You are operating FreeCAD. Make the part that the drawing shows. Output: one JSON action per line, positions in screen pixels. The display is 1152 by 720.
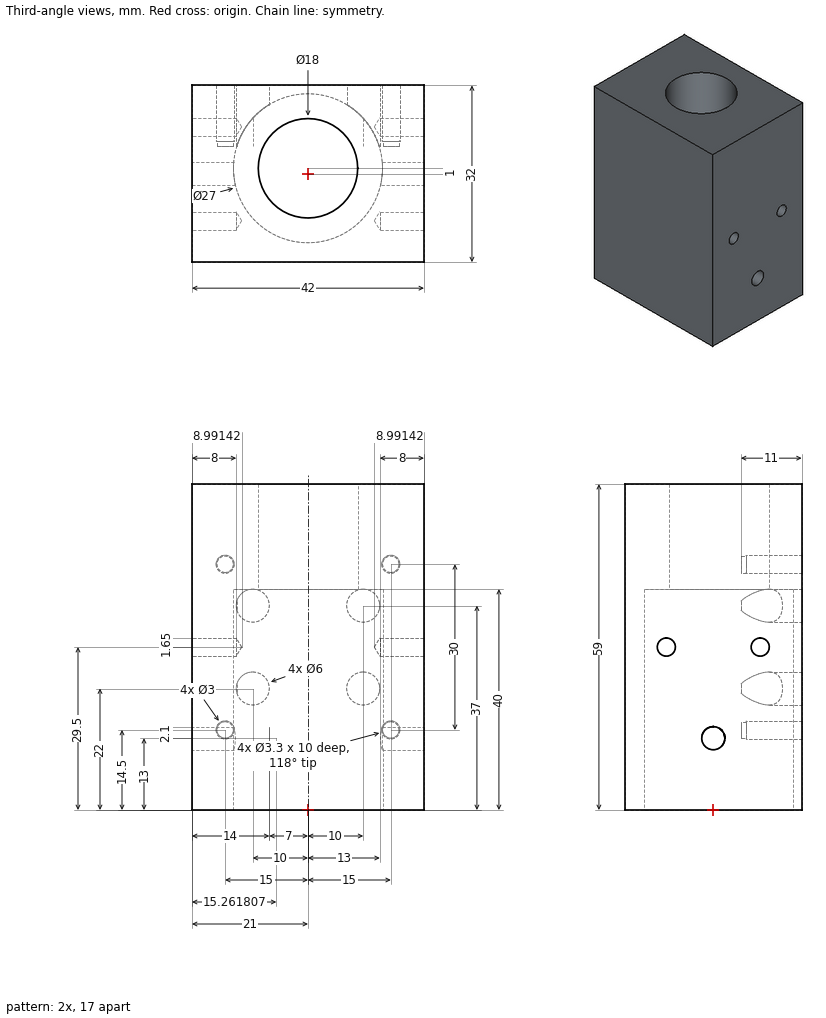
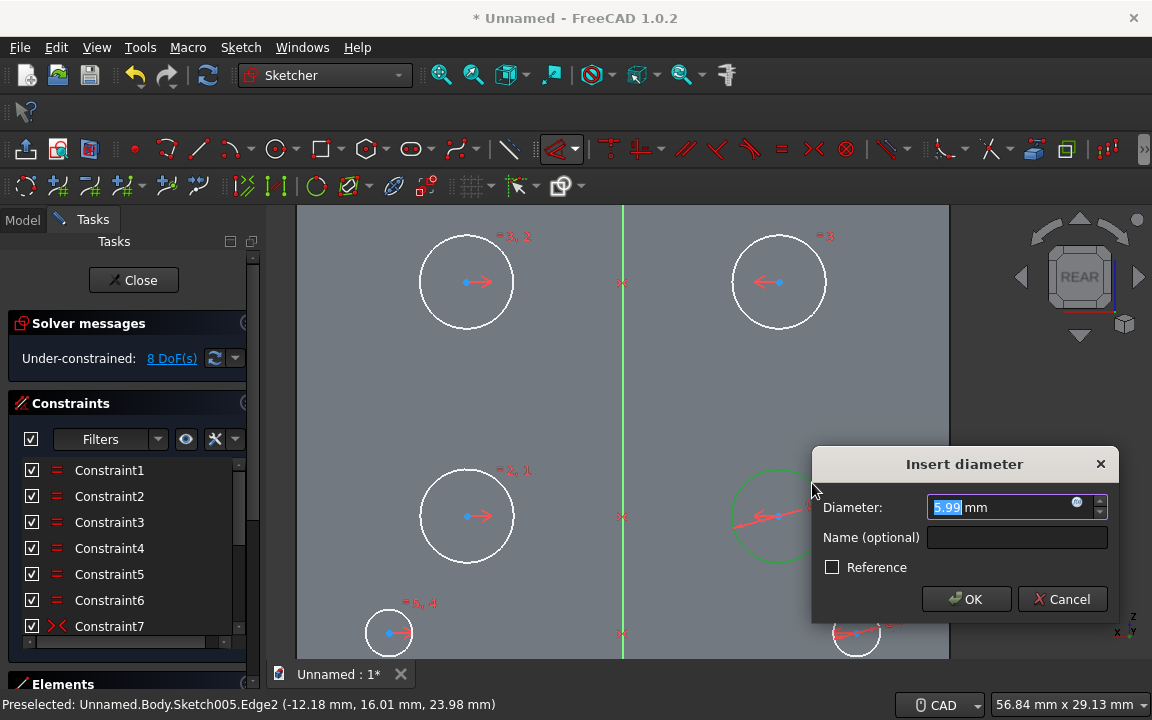
{"action": "type", "text": "6"}
{"action": "key", "text": "Return"}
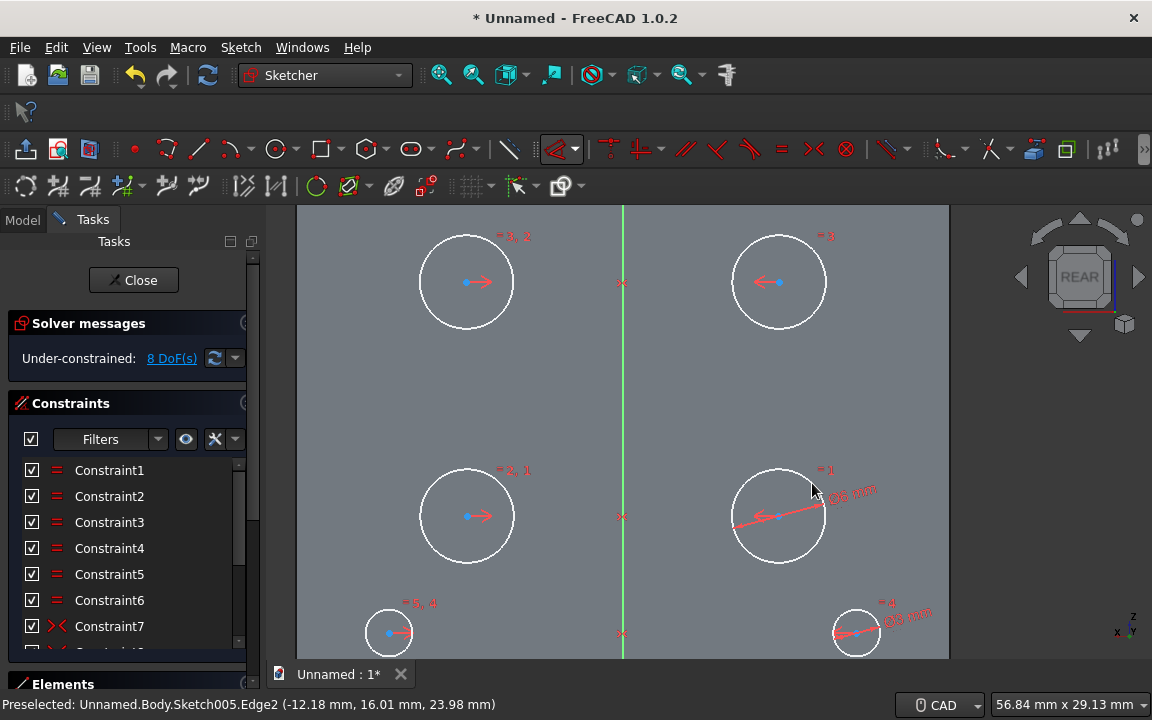
{"action": "scroll", "coordinate": [651, 393], "scroll_direction": "down", "scroll_amount": 5}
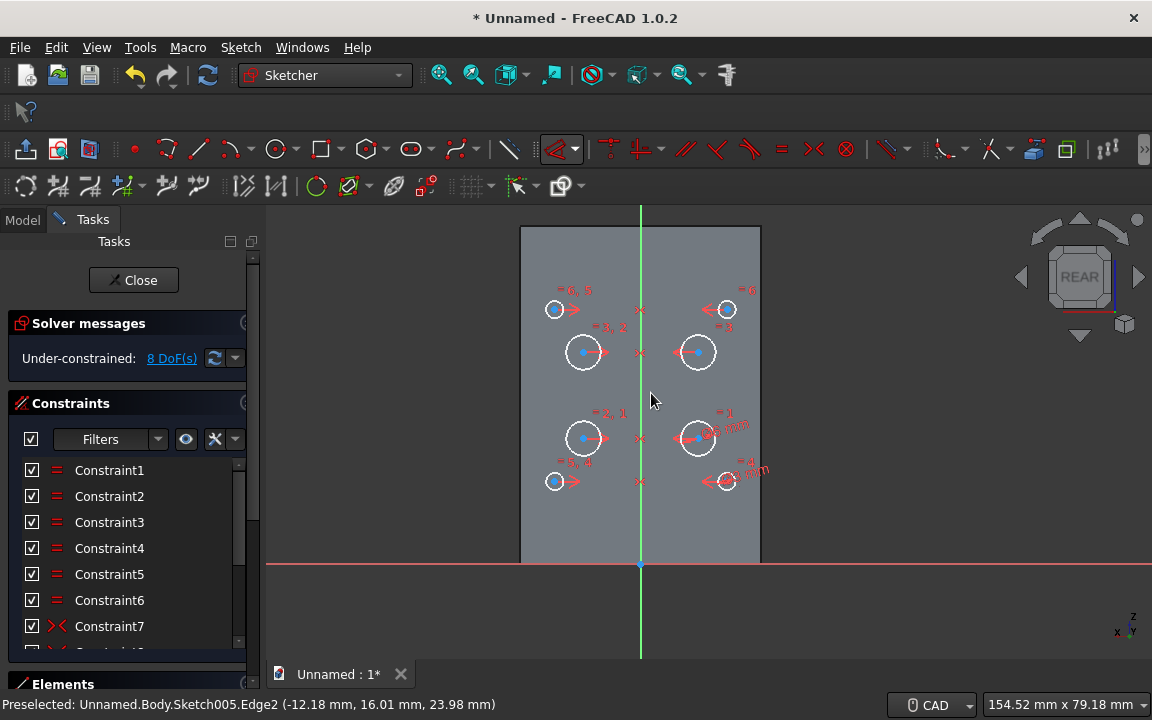
{"action": "left_click", "coordinate": [727, 482]}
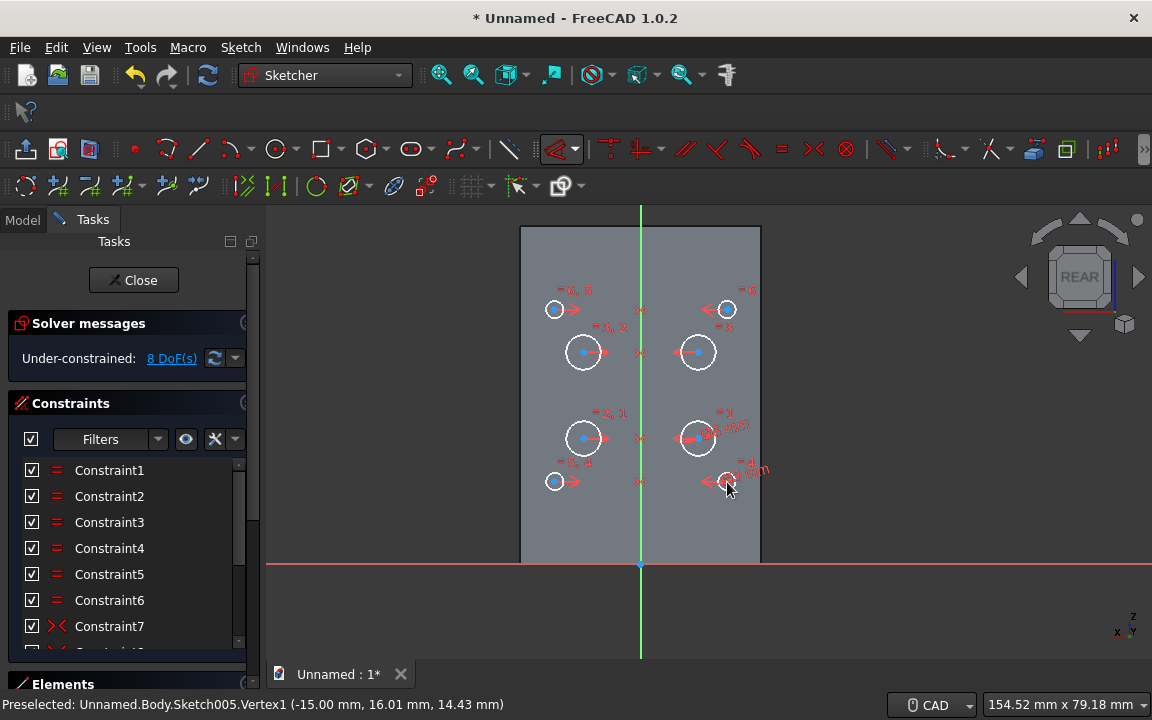
{"action": "key", "text": "l"}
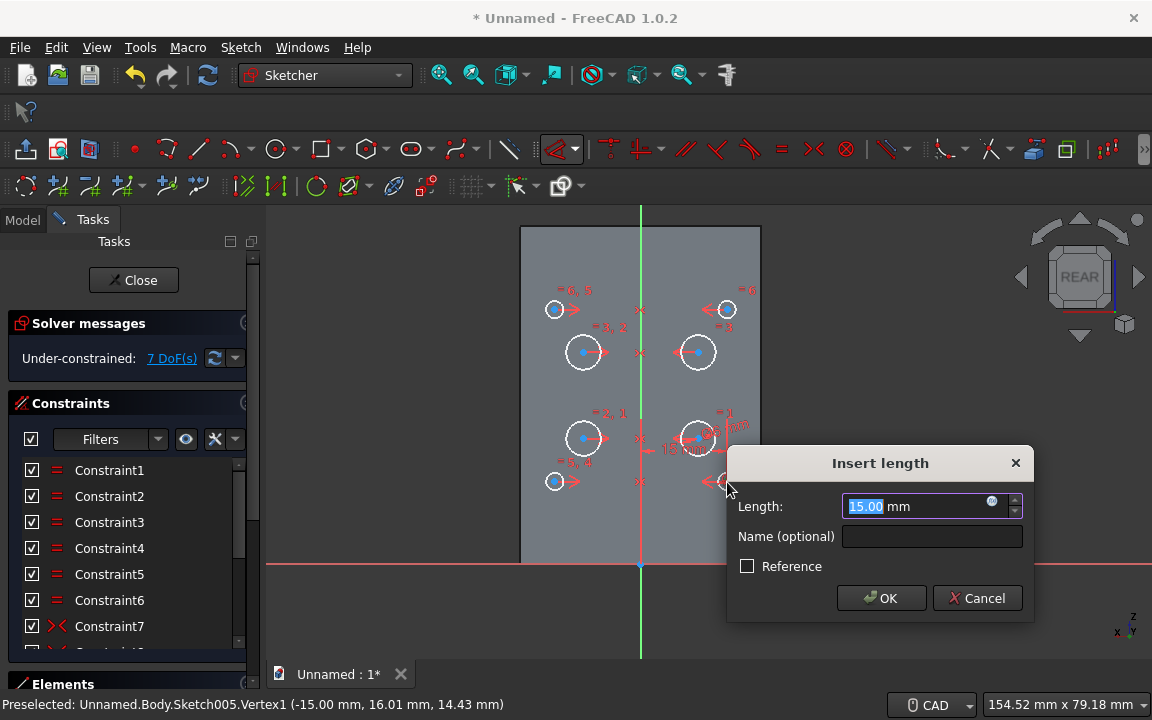
{"action": "type", "text": "15"}
{"action": "key", "text": "Return"}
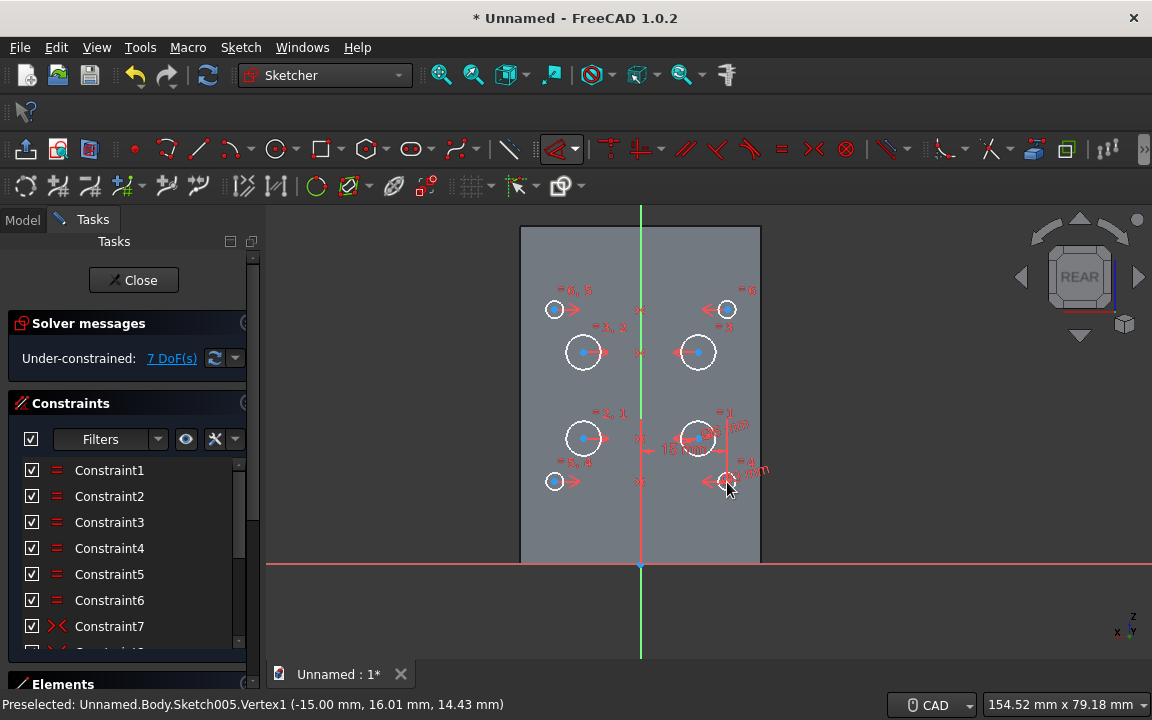
{"action": "left_click", "coordinate": [698, 439]}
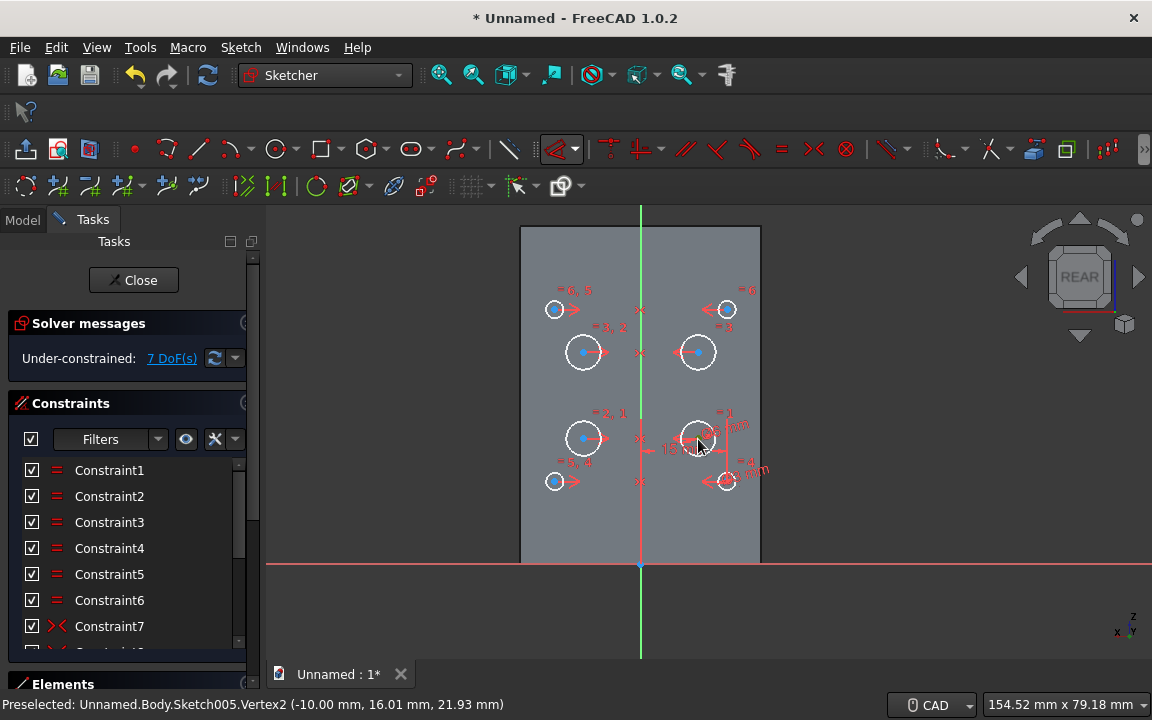
{"action": "key", "text": "l"}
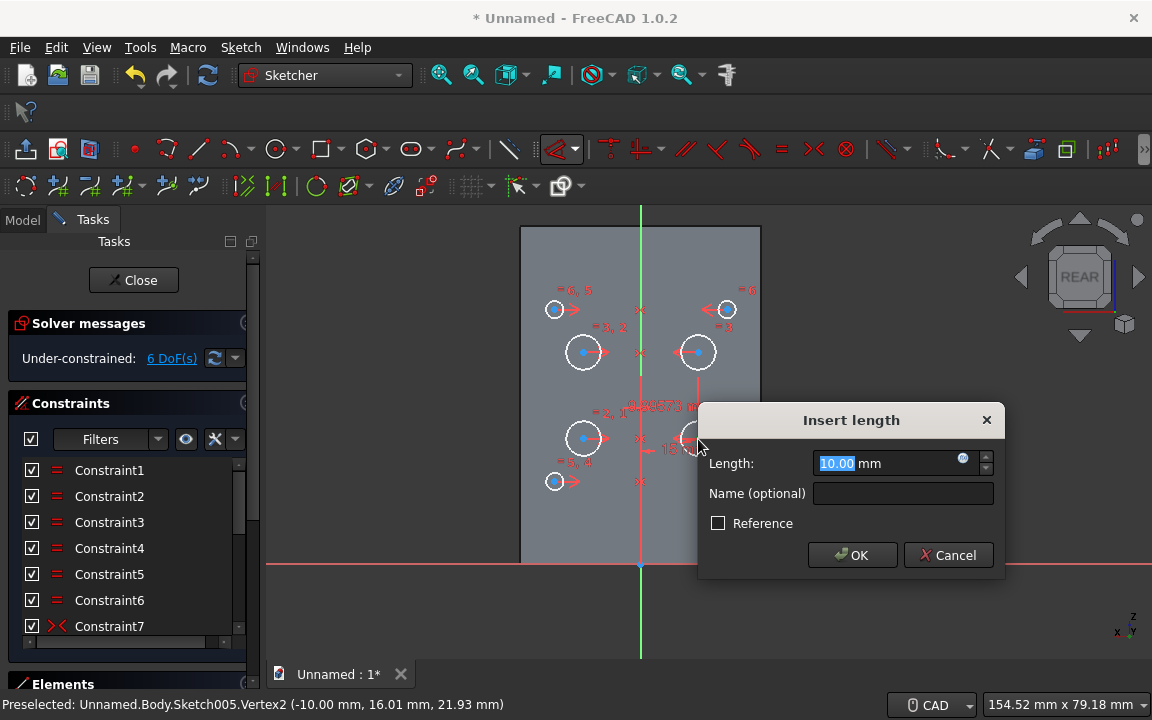
{"action": "type", "text": "10"}
{"action": "key", "text": "Return"}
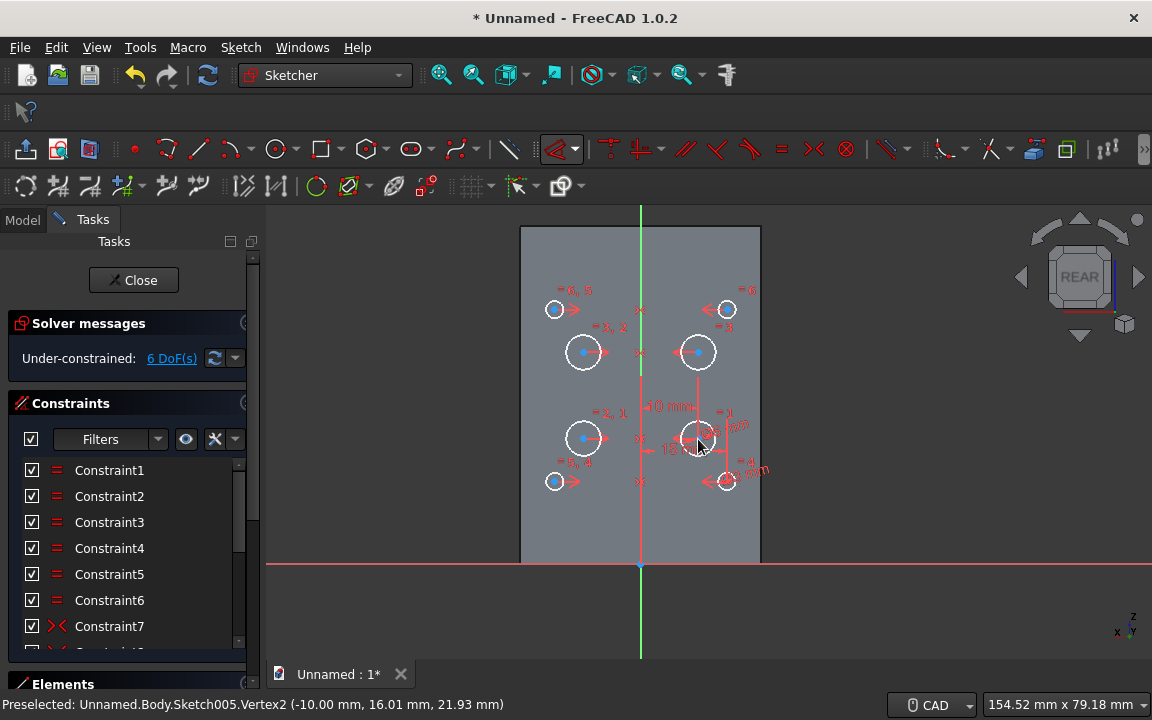
{"action": "left_click", "coordinate": [698, 439]}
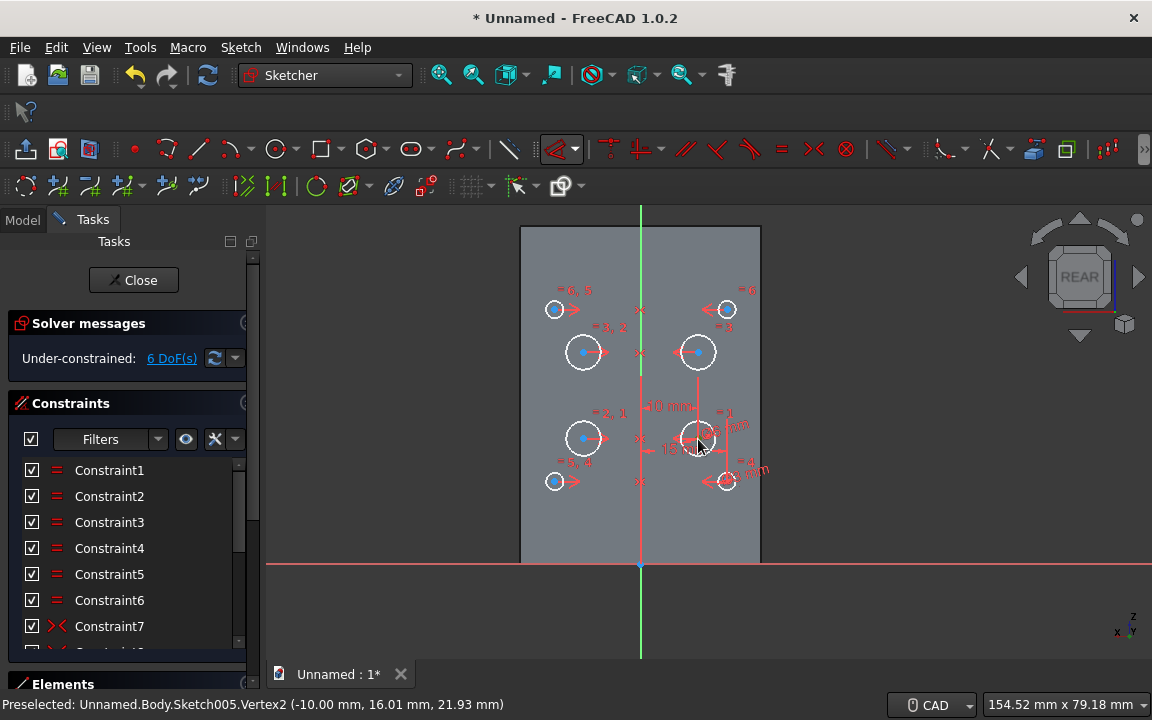
{"action": "left_click", "coordinate": [578, 150]}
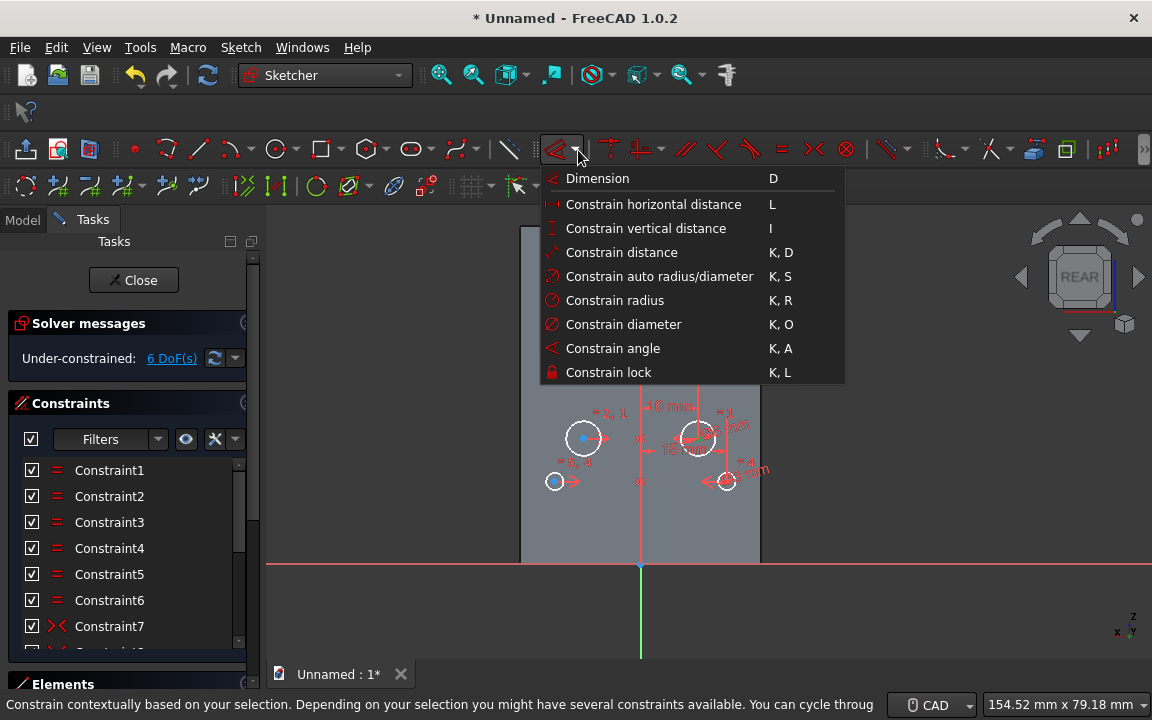
{"action": "left_click", "coordinate": [693, 228]}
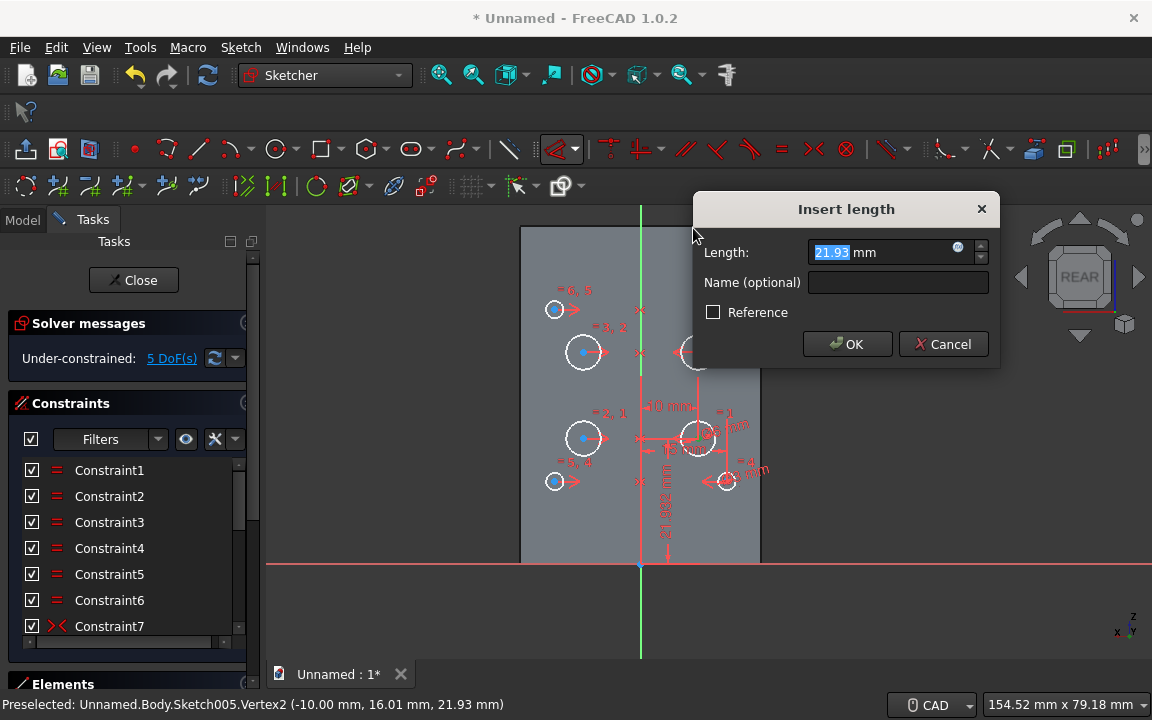
{"action": "type", "text": "22"}
{"action": "key", "text": "Return"}